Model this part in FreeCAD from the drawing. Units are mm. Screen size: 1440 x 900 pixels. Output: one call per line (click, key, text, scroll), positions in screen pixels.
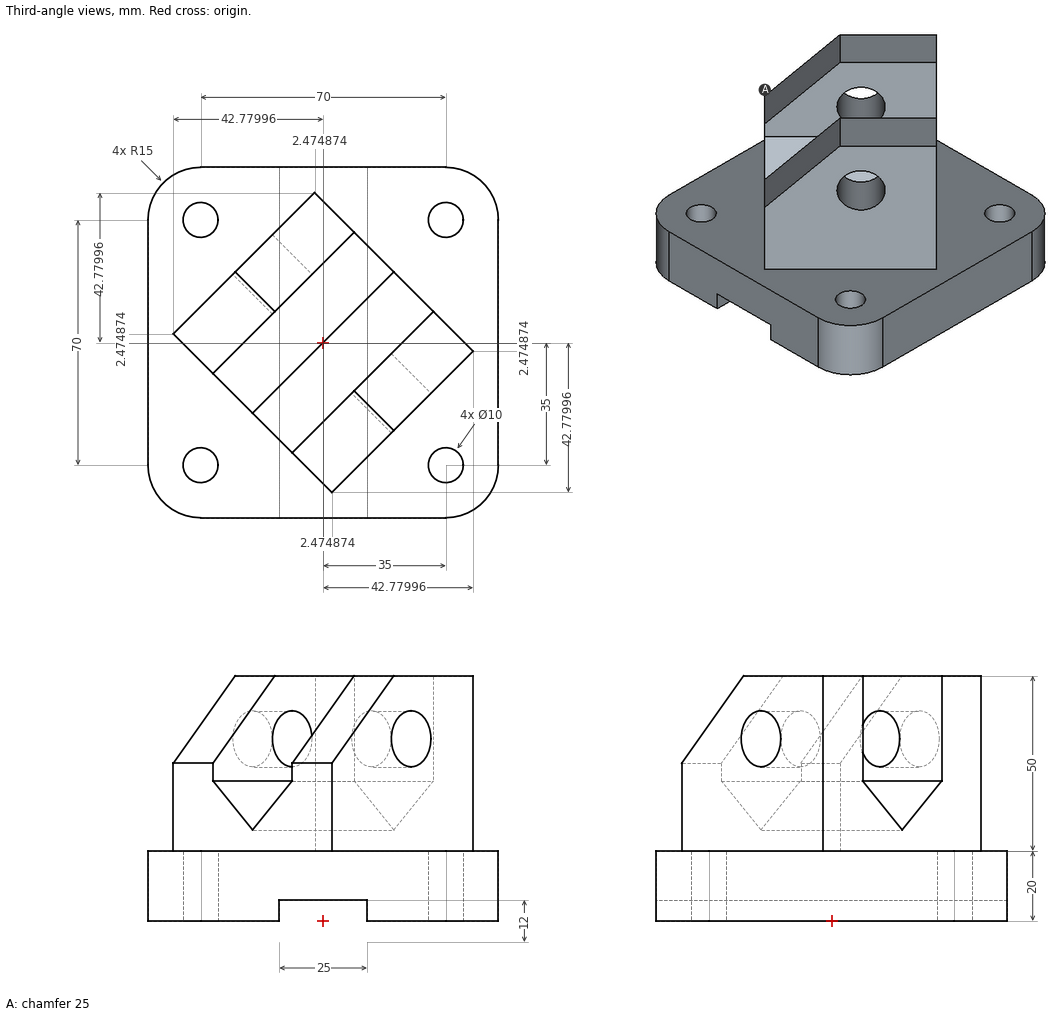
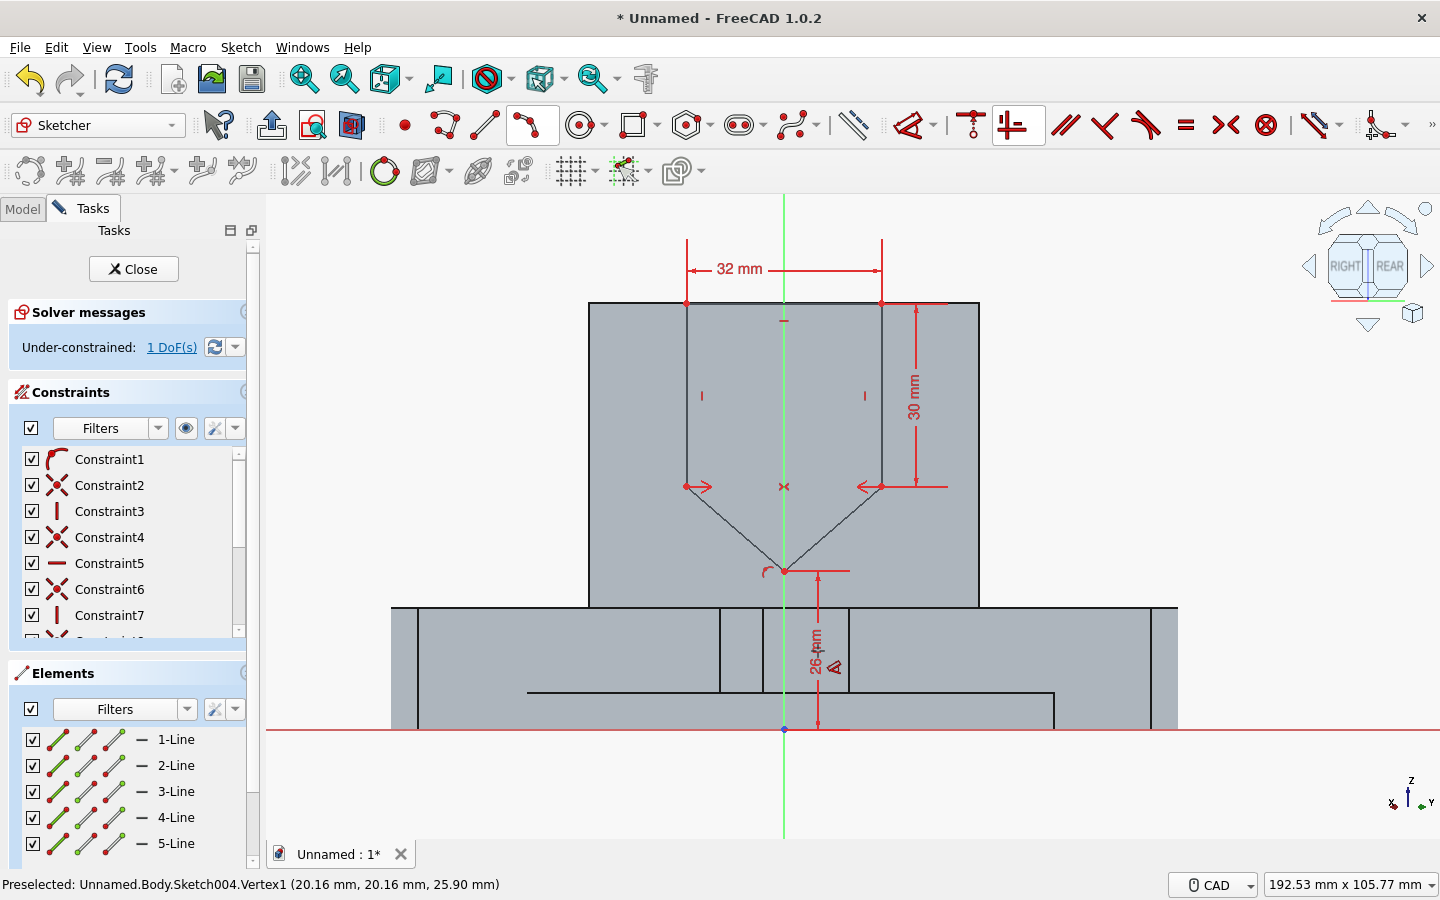
click(882, 487)
click(916, 608)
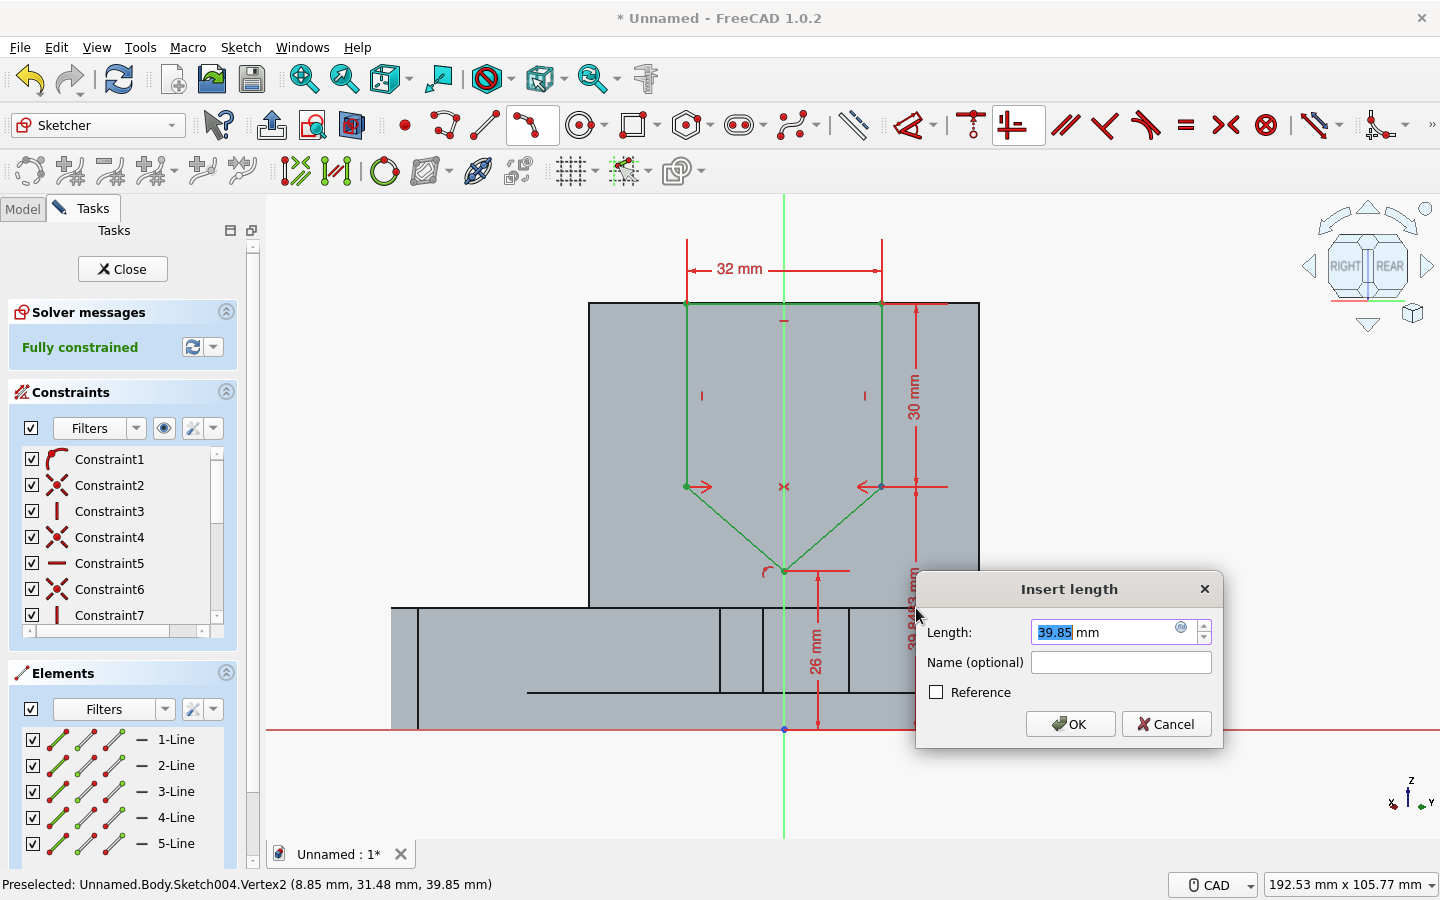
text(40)
key(Return)
key(Escape)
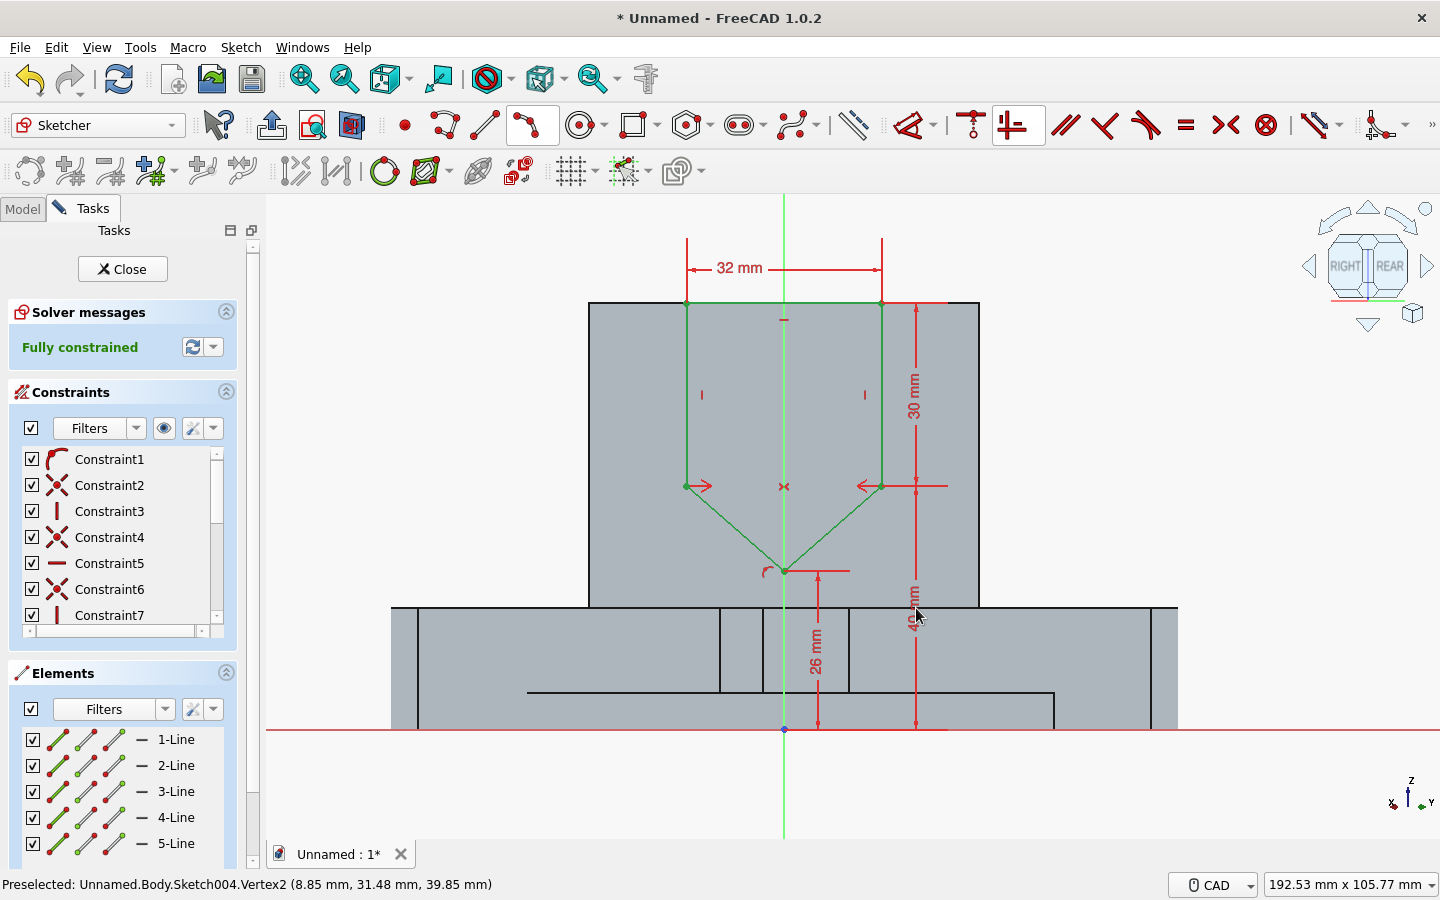
click(123, 269)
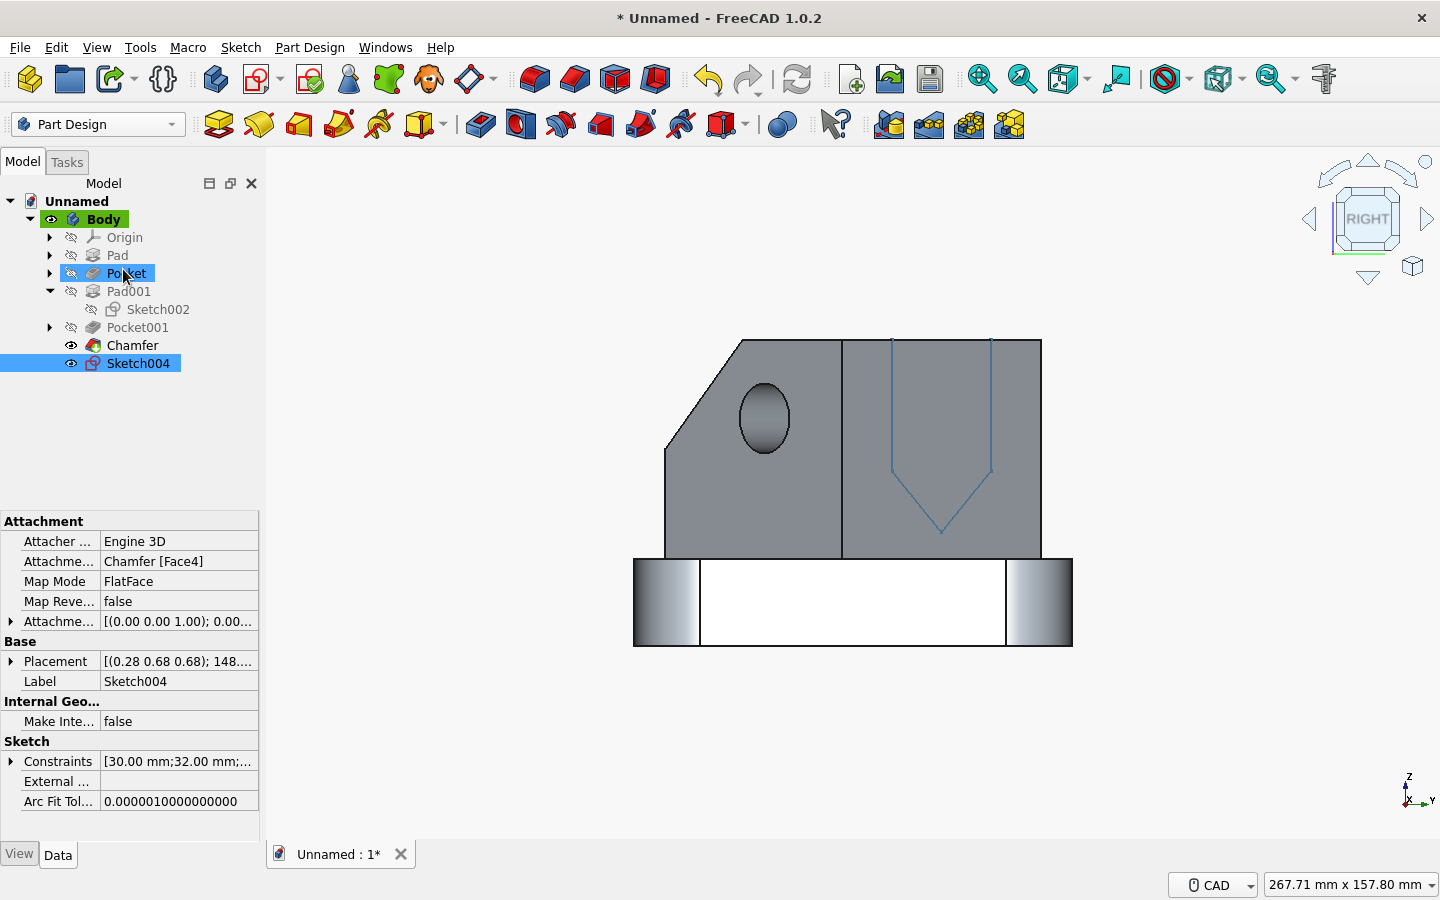
click(482, 124)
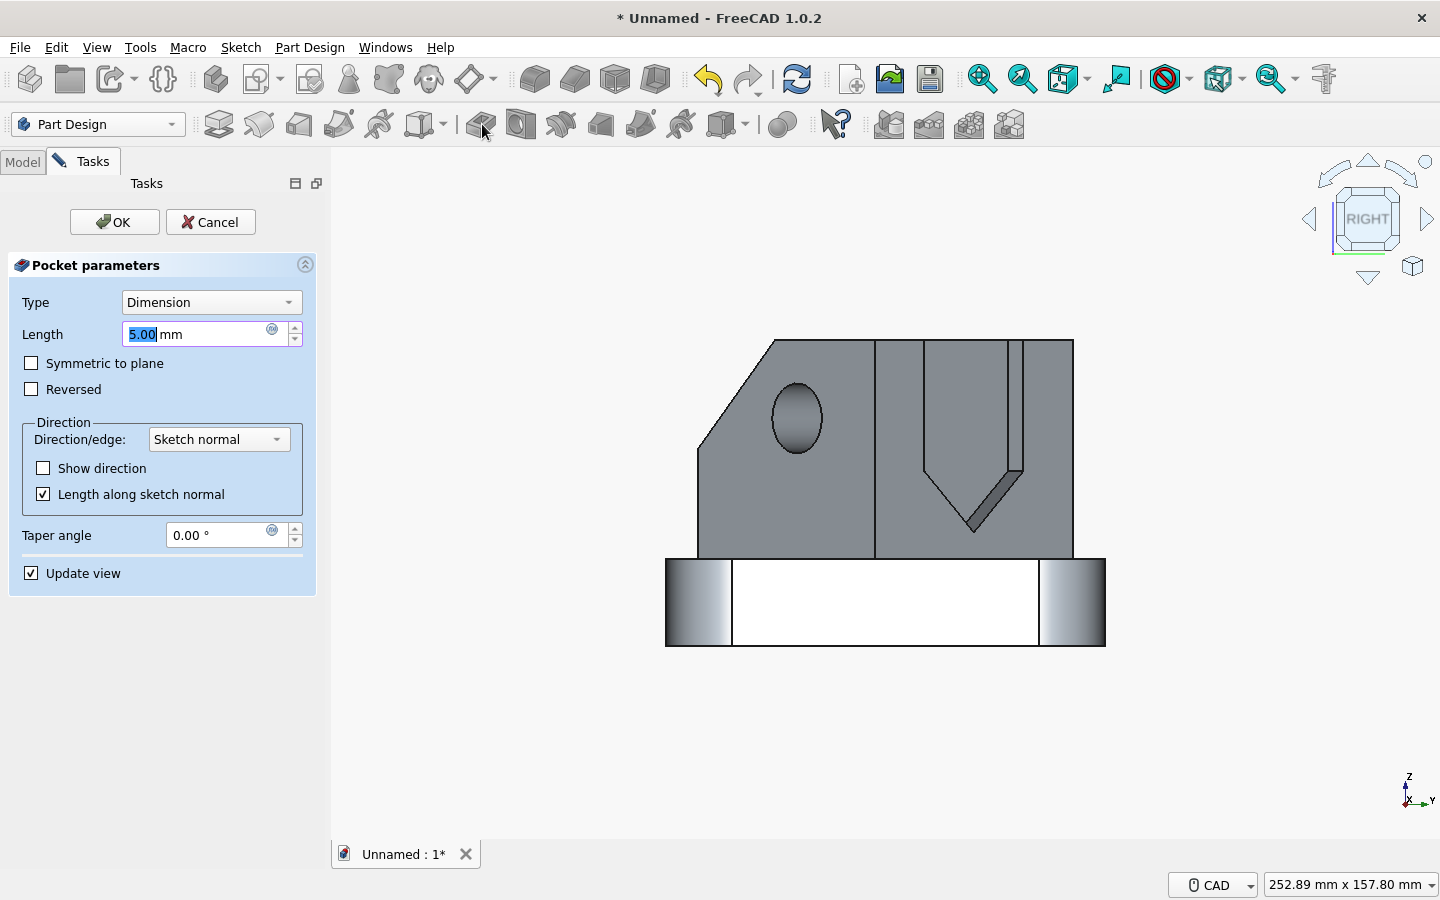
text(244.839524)
key(Tab)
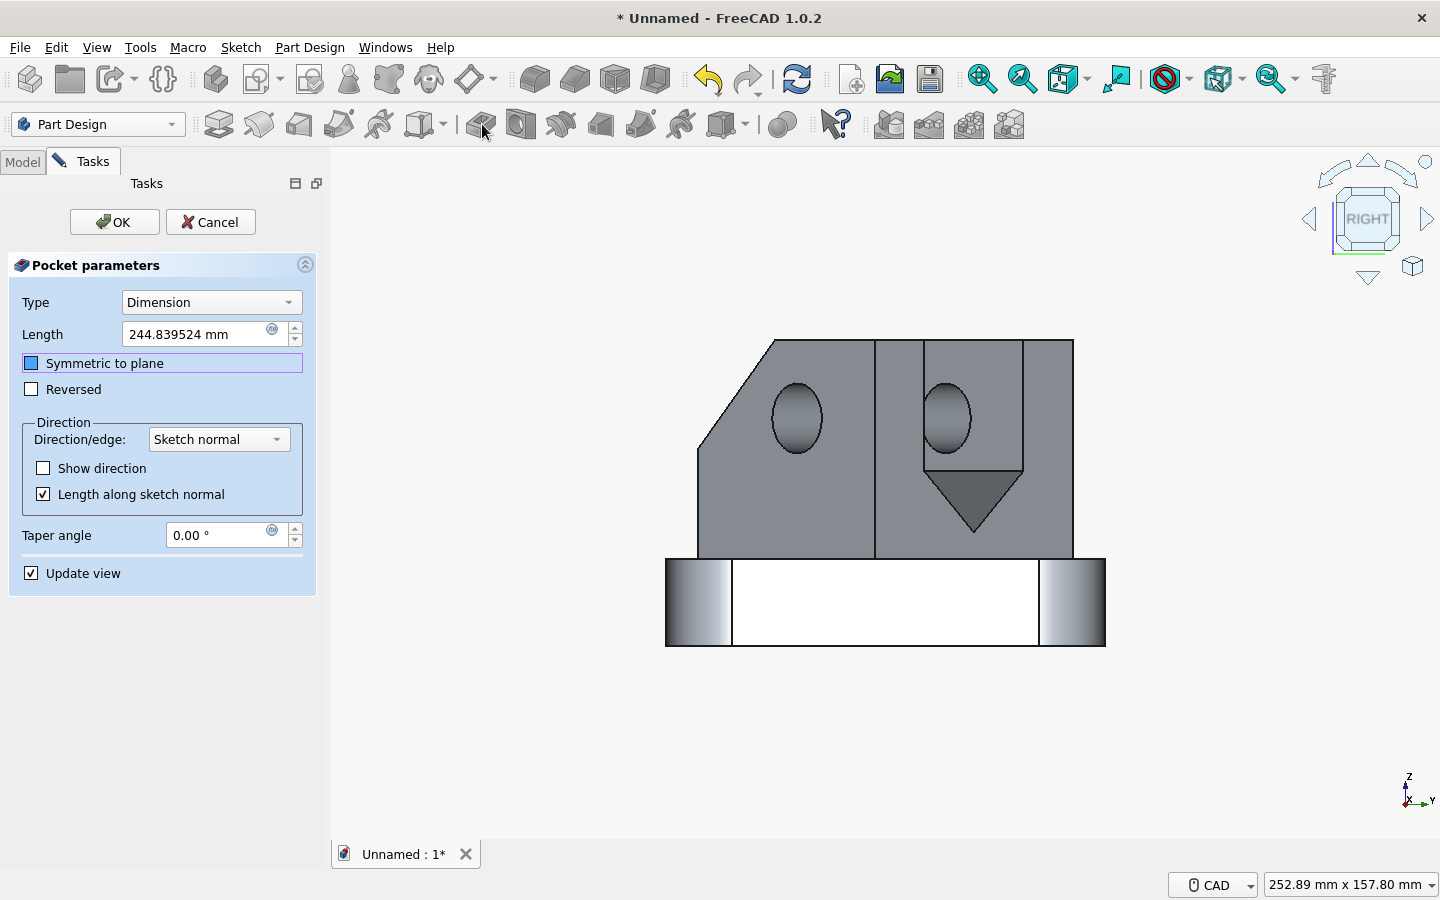
click(30, 363)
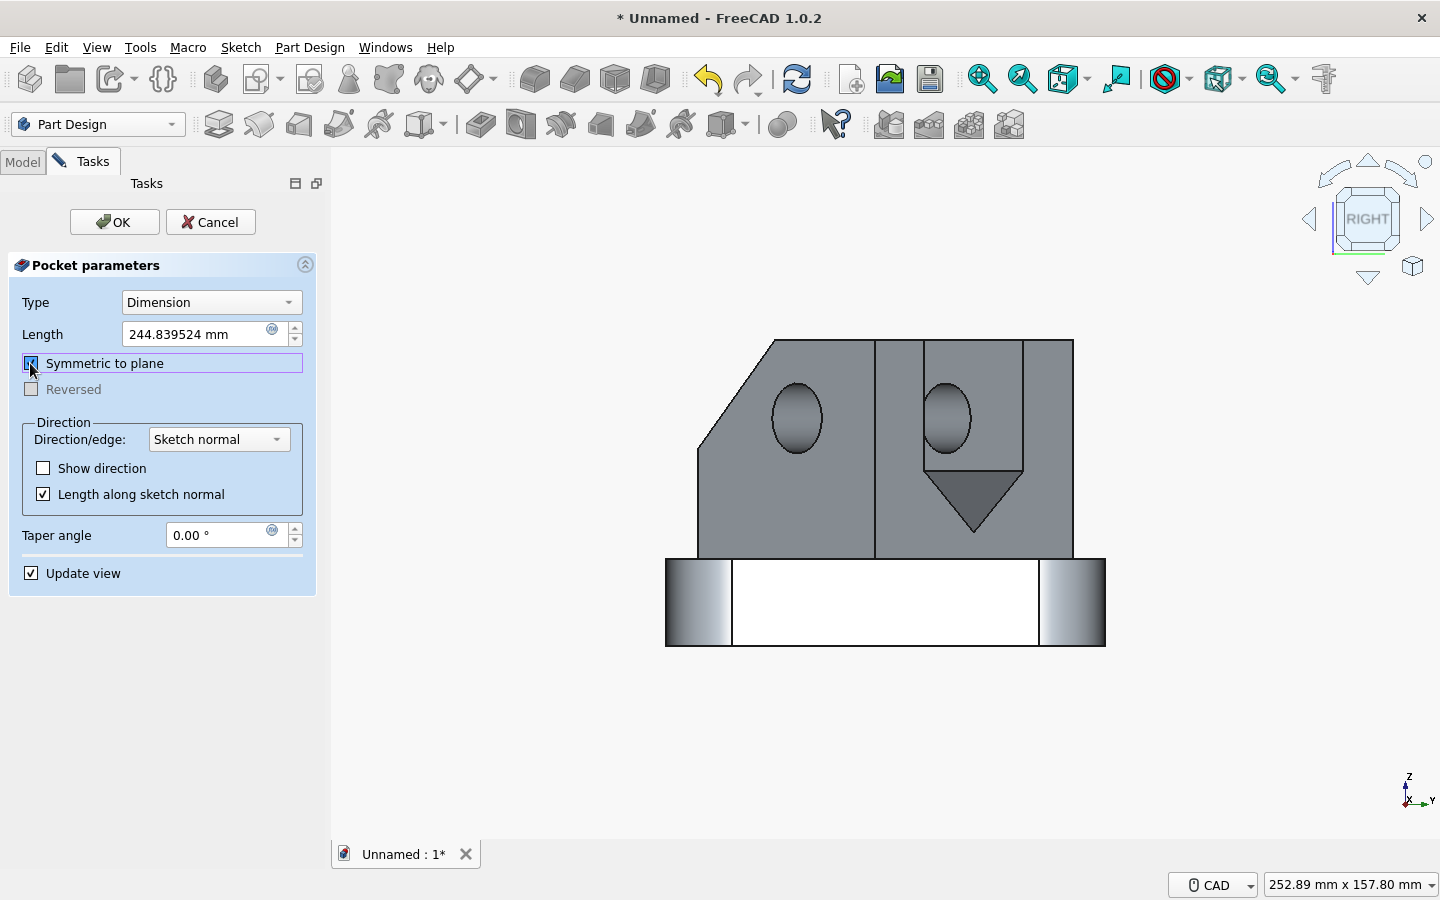
click(115, 222)